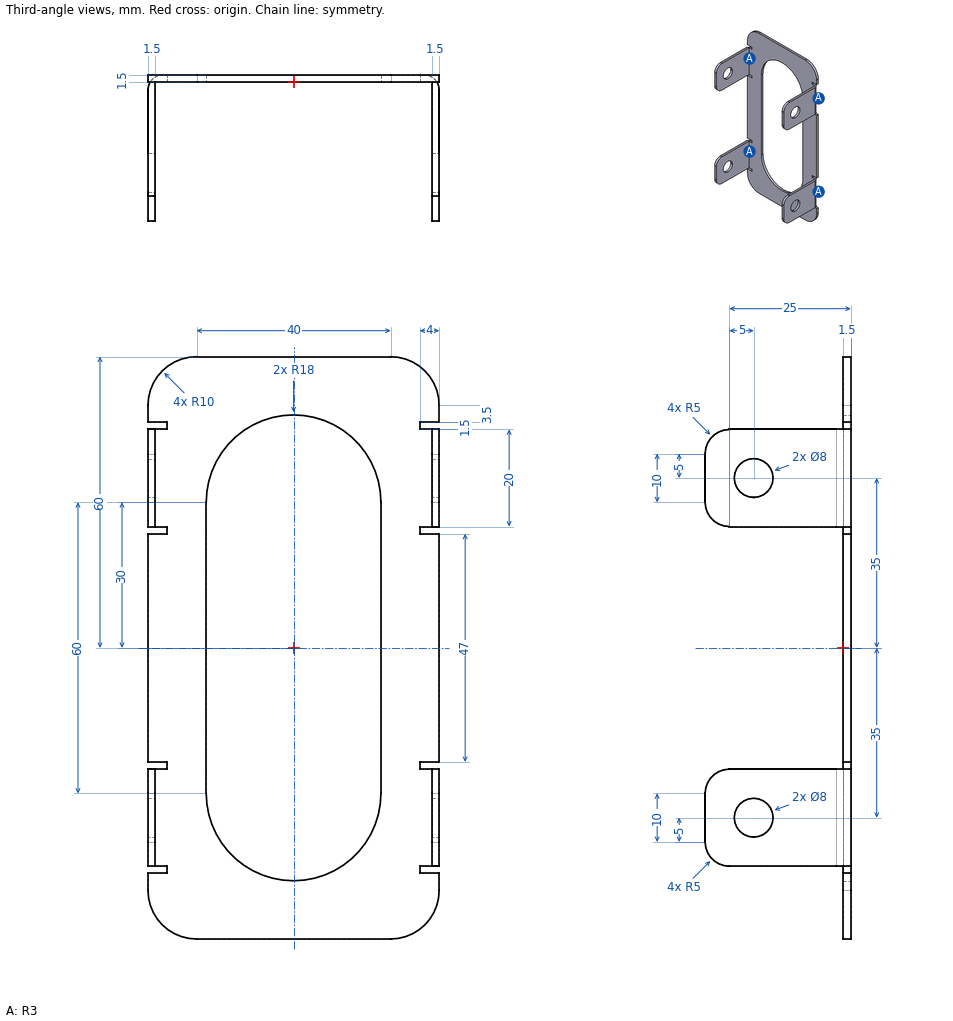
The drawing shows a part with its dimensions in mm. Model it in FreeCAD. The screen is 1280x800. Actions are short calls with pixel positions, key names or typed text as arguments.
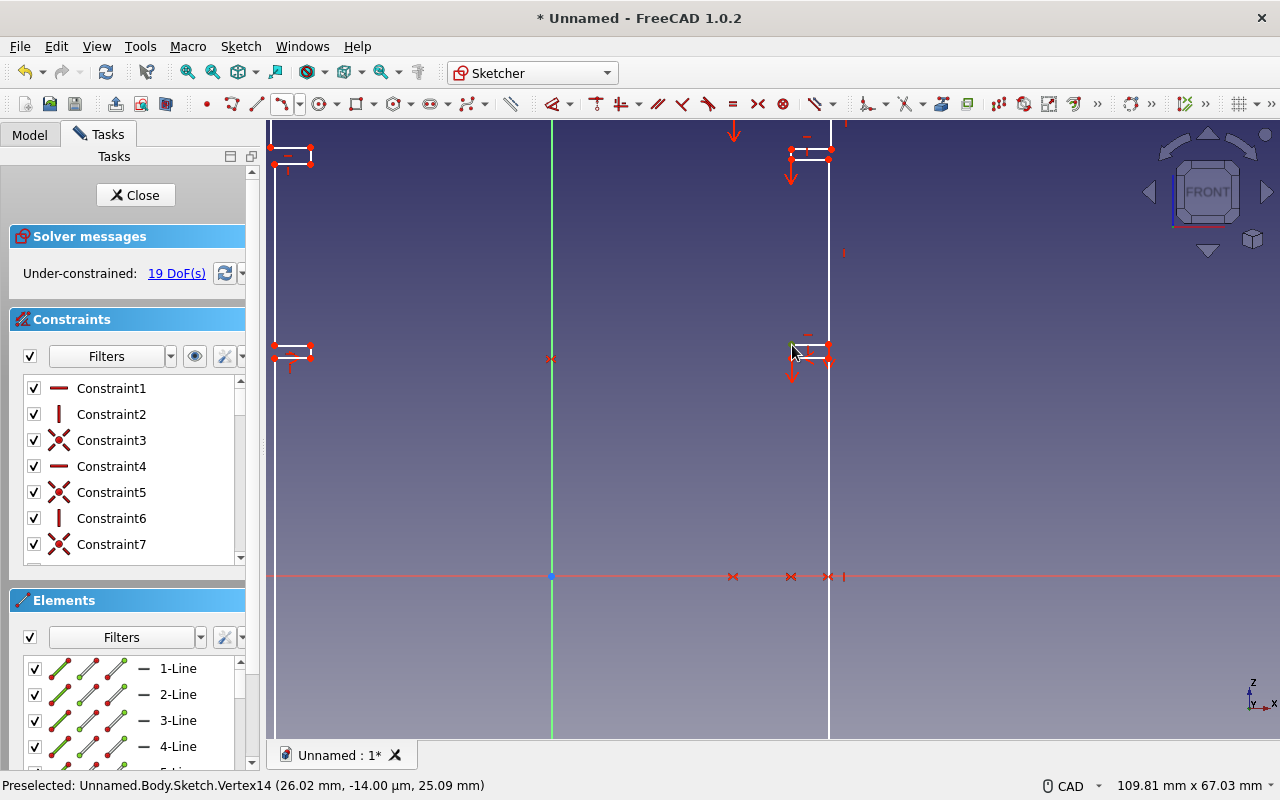
click(311, 346)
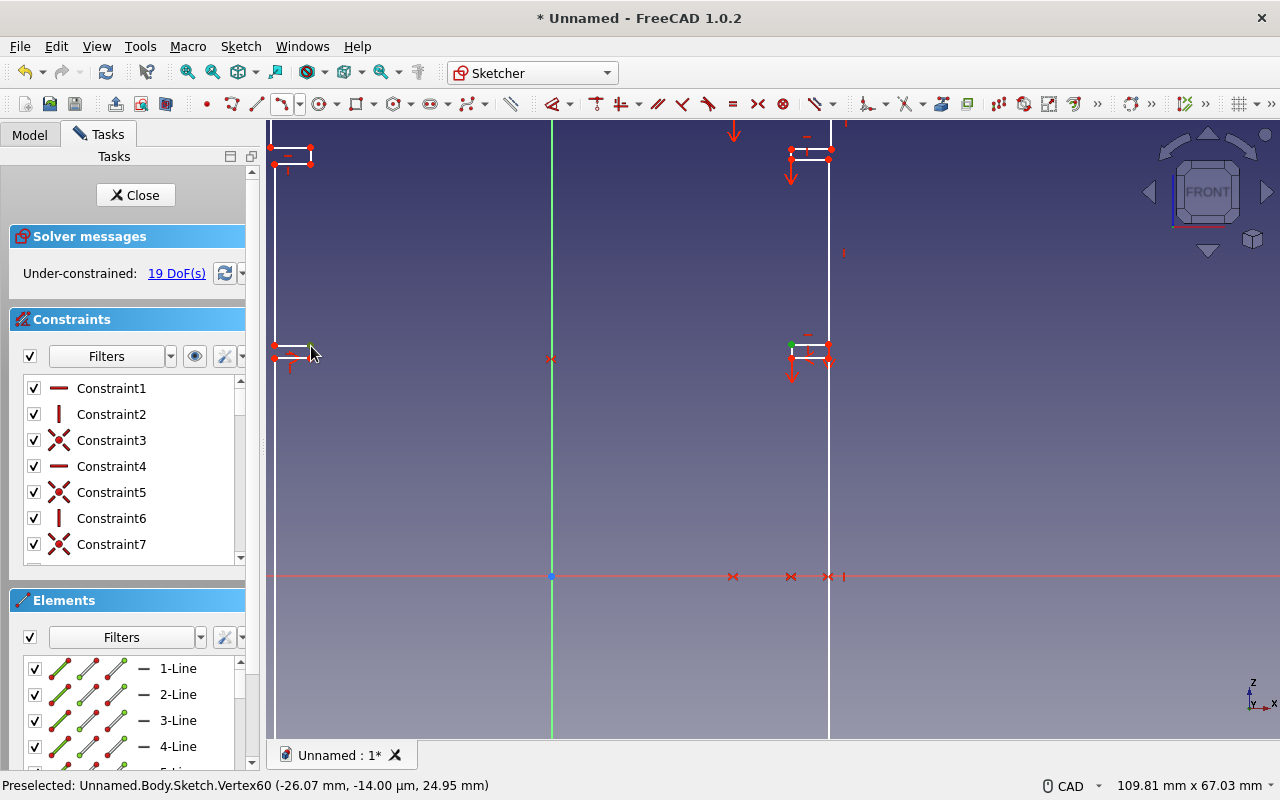
click(552, 671)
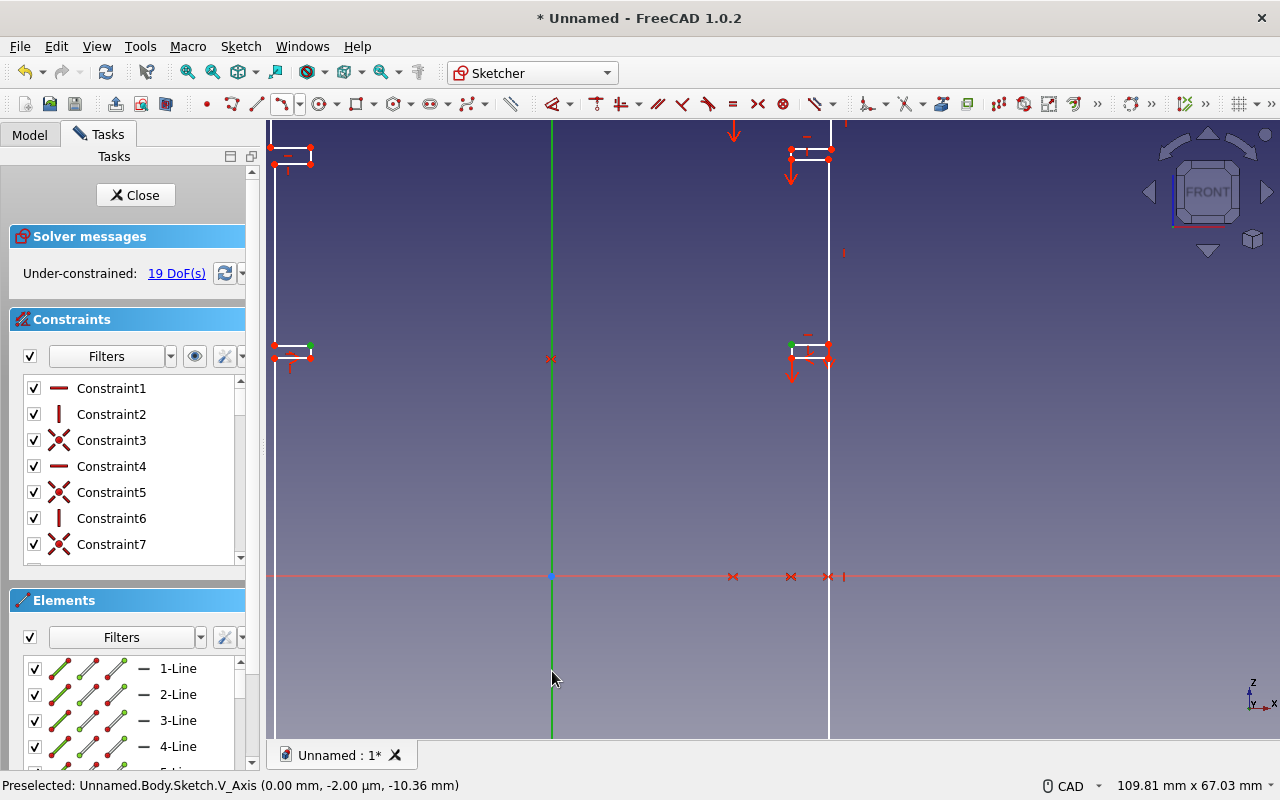
click(758, 104)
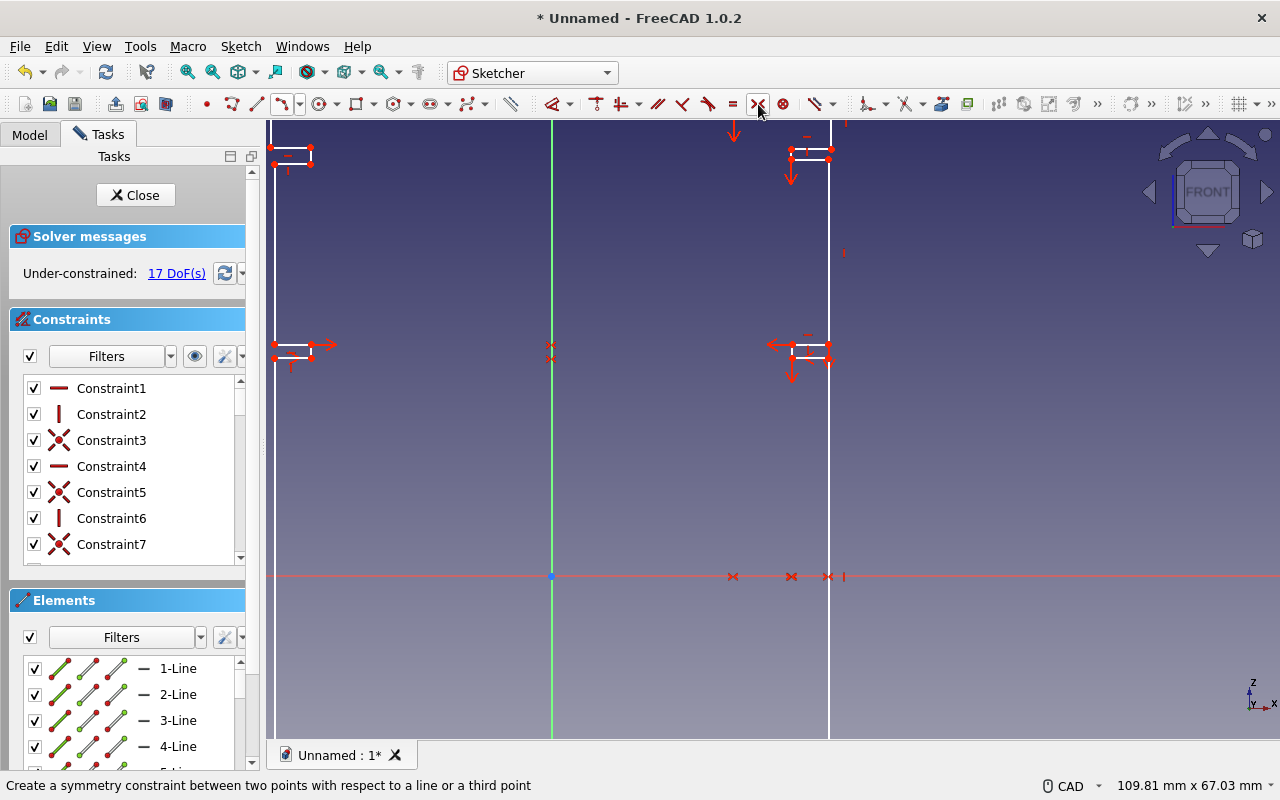
click(829, 160)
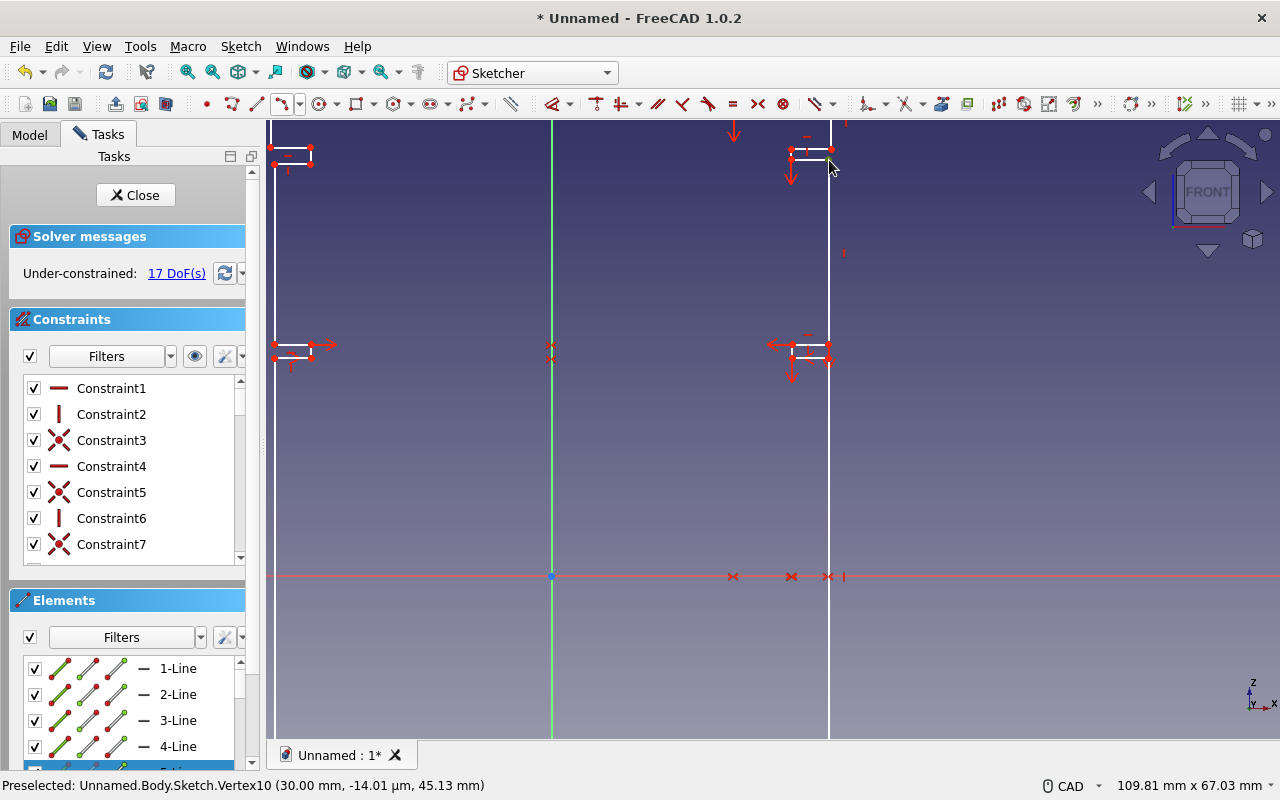
scroll(793, 344, down, 5)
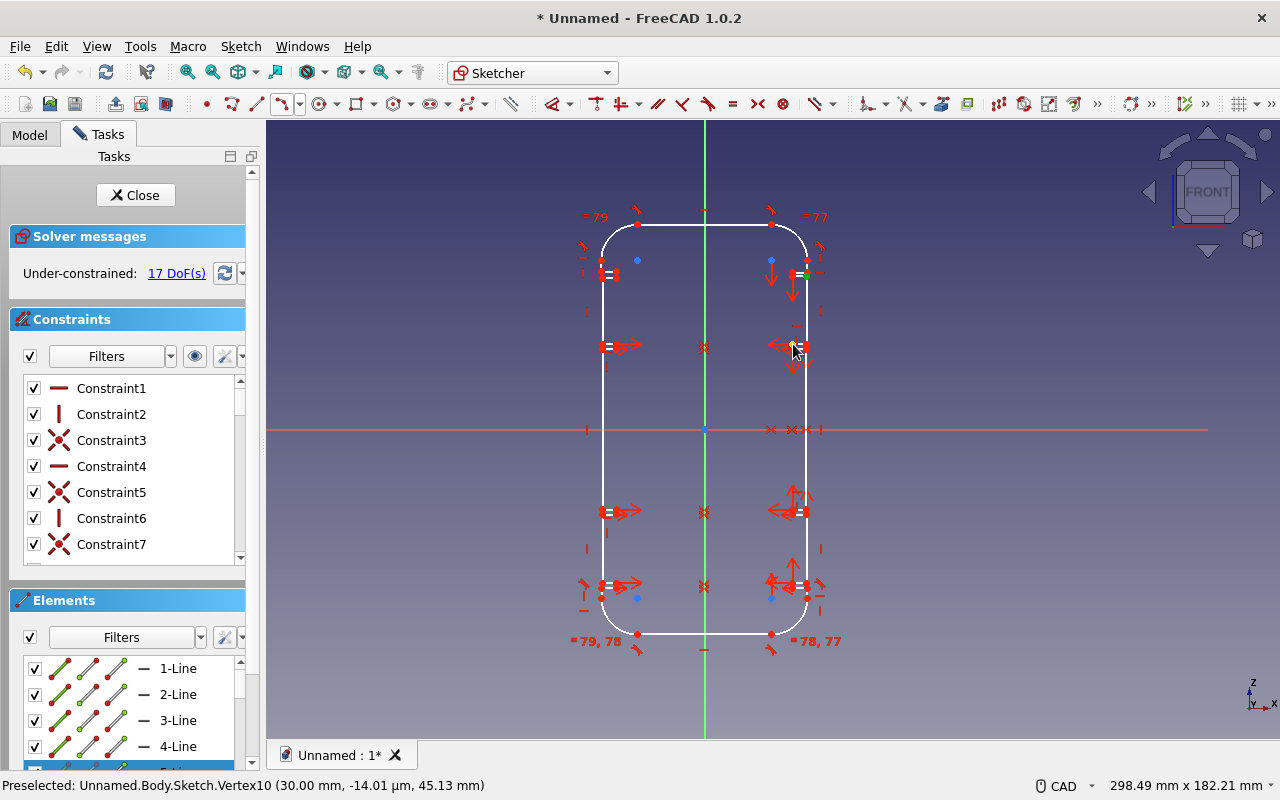
scroll(603, 278, up, 4)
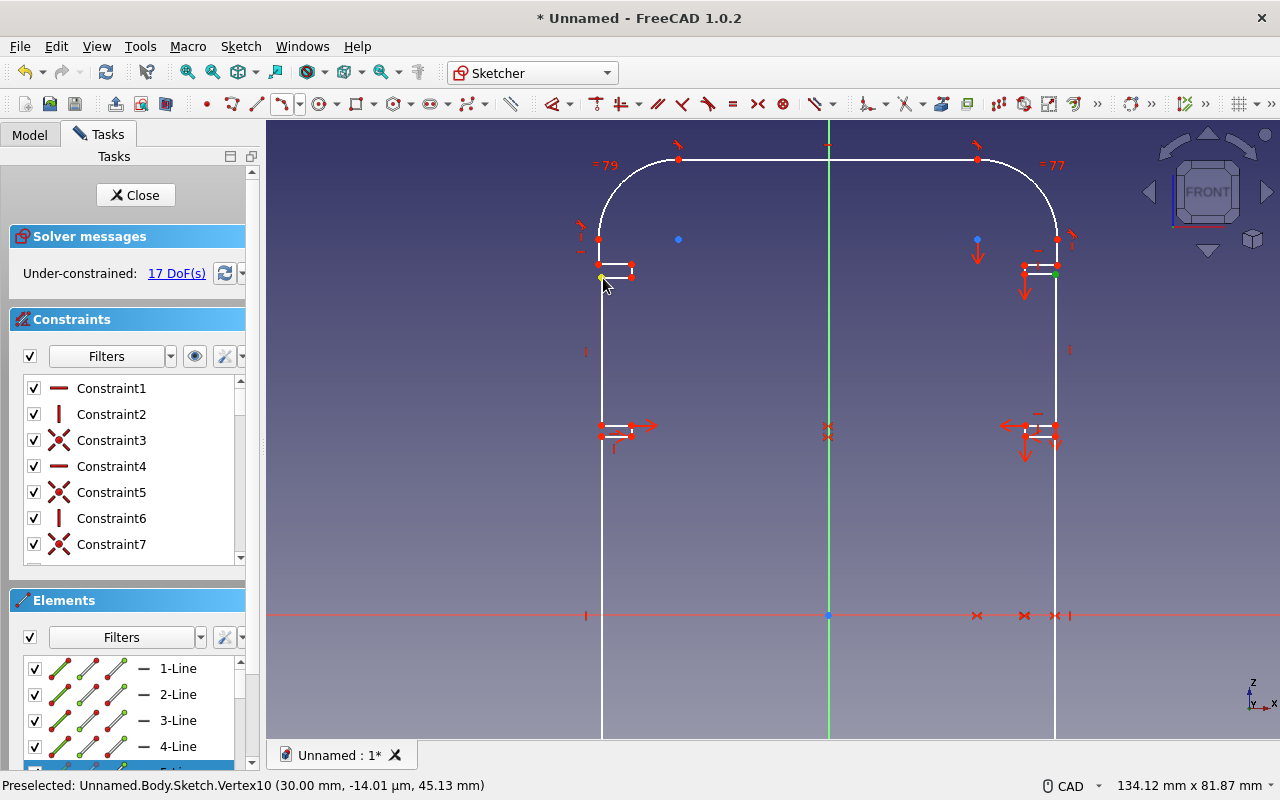
click(602, 278)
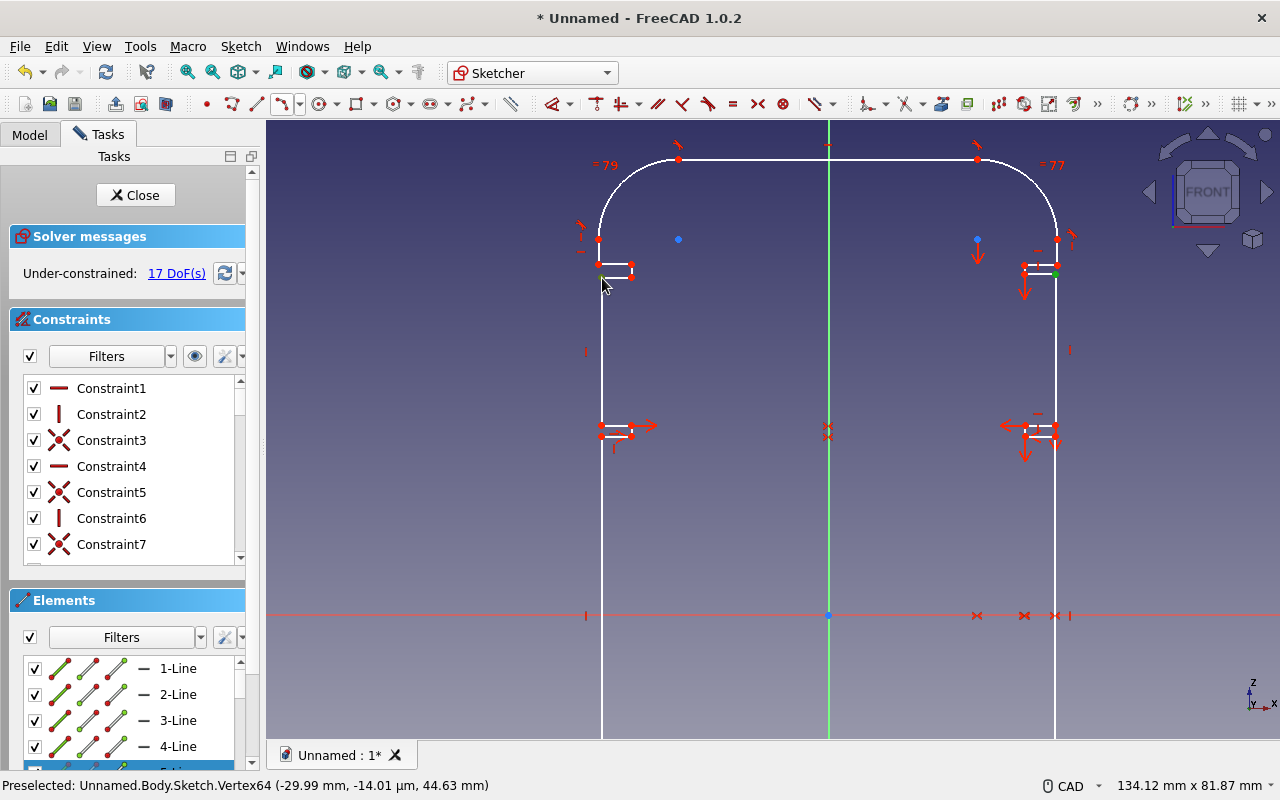
click(829, 671)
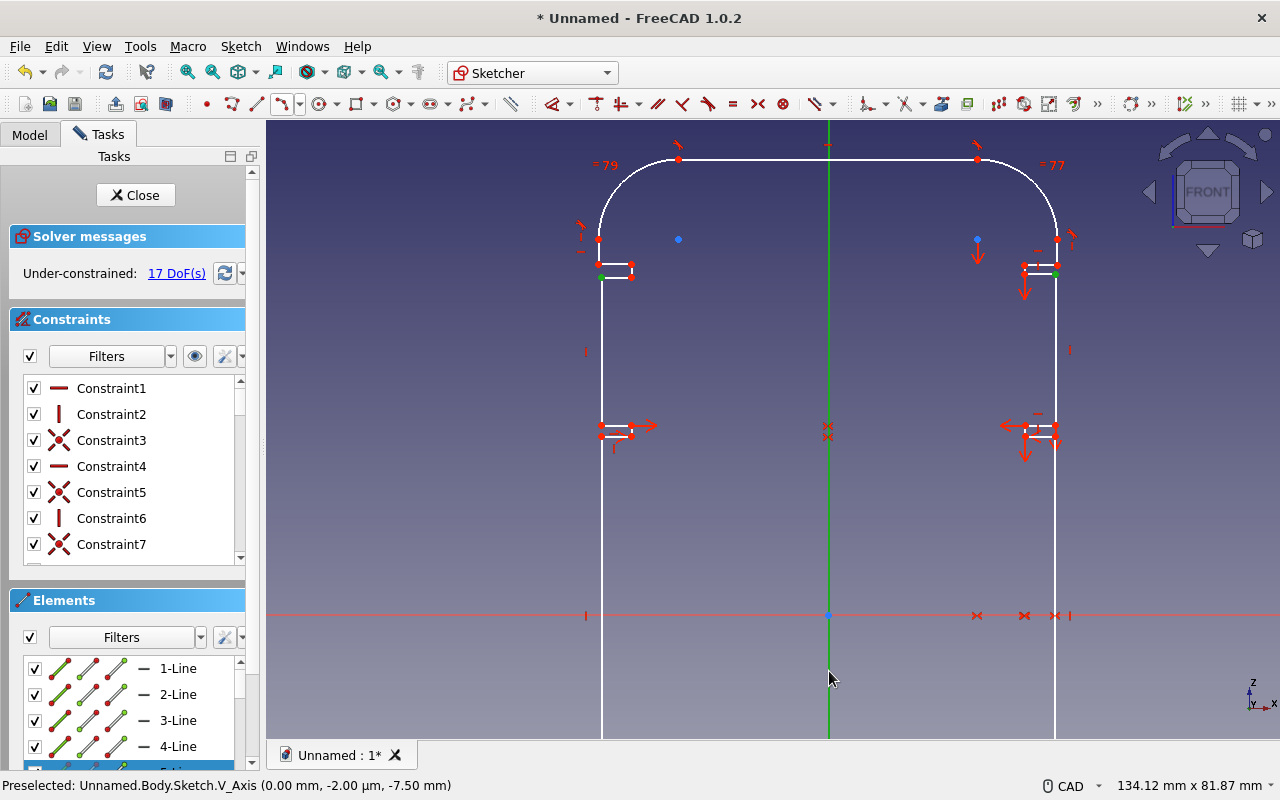
click(758, 104)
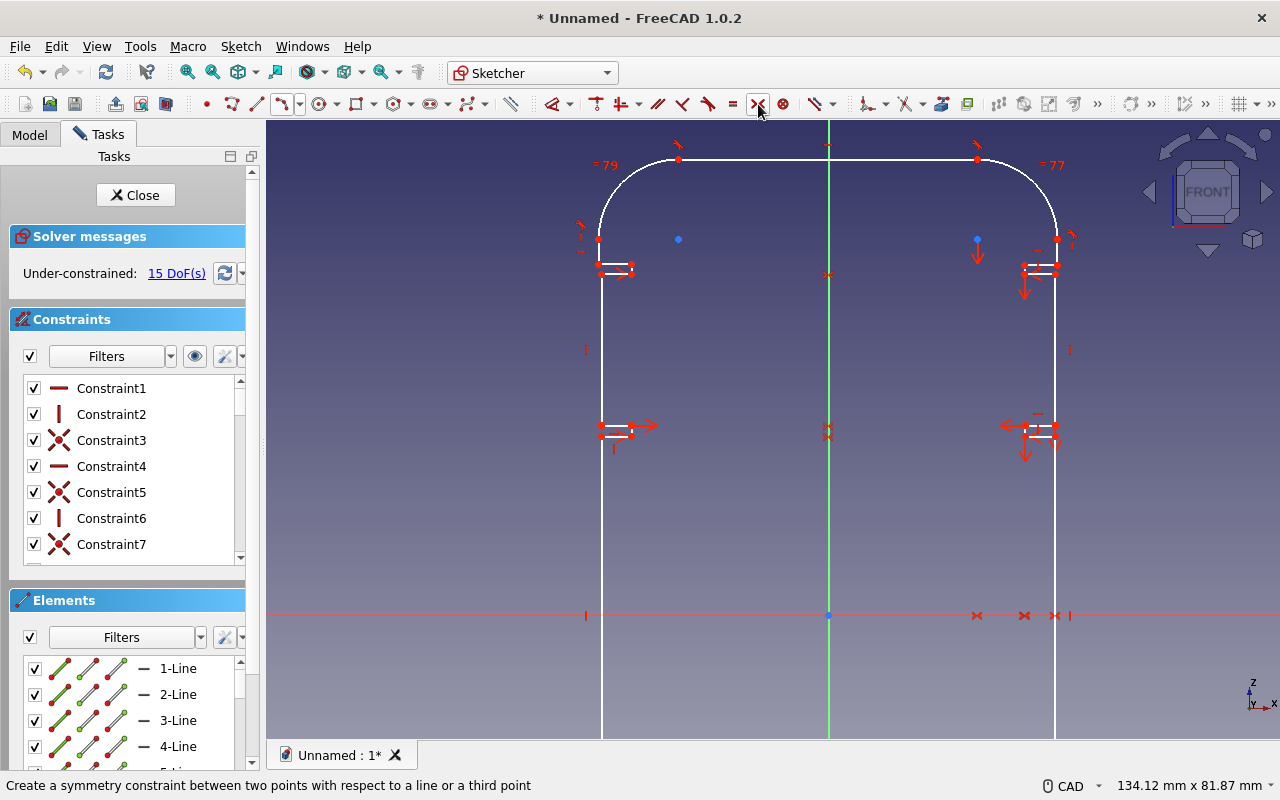
scroll(1025, 265, up, 2)